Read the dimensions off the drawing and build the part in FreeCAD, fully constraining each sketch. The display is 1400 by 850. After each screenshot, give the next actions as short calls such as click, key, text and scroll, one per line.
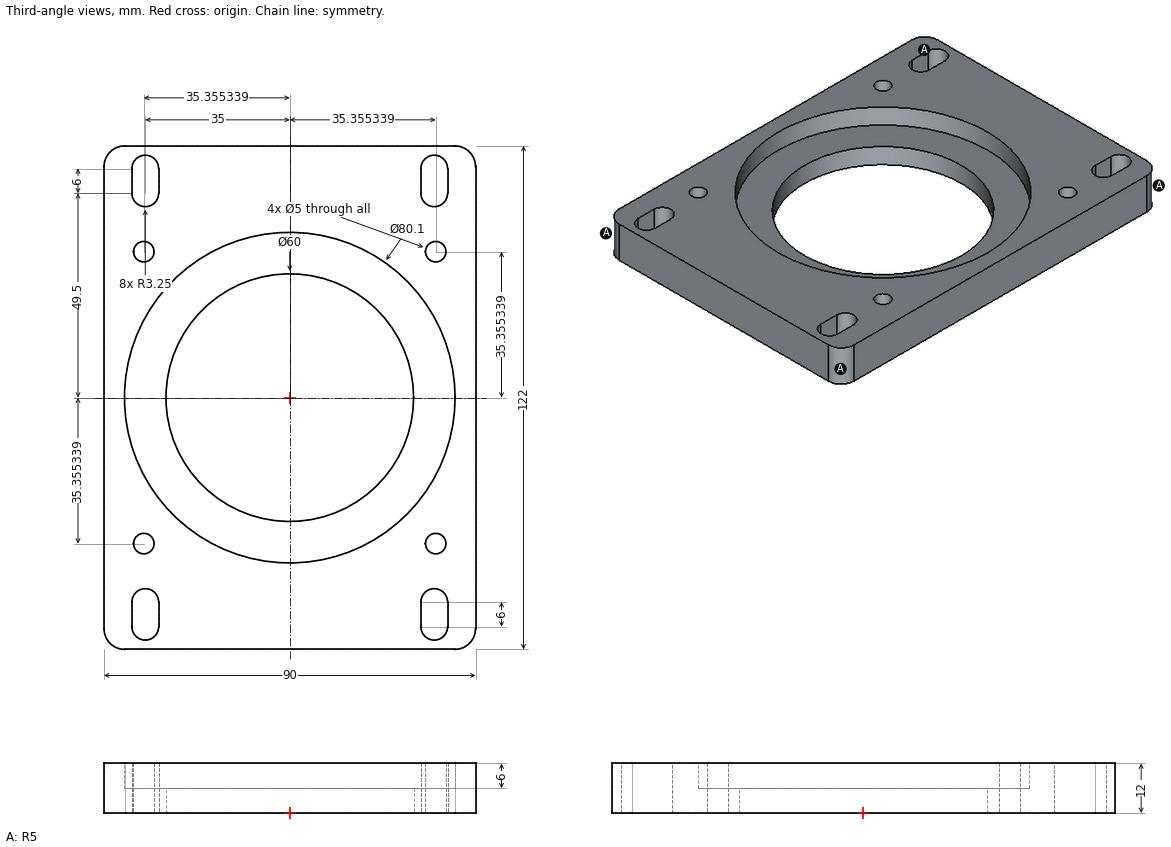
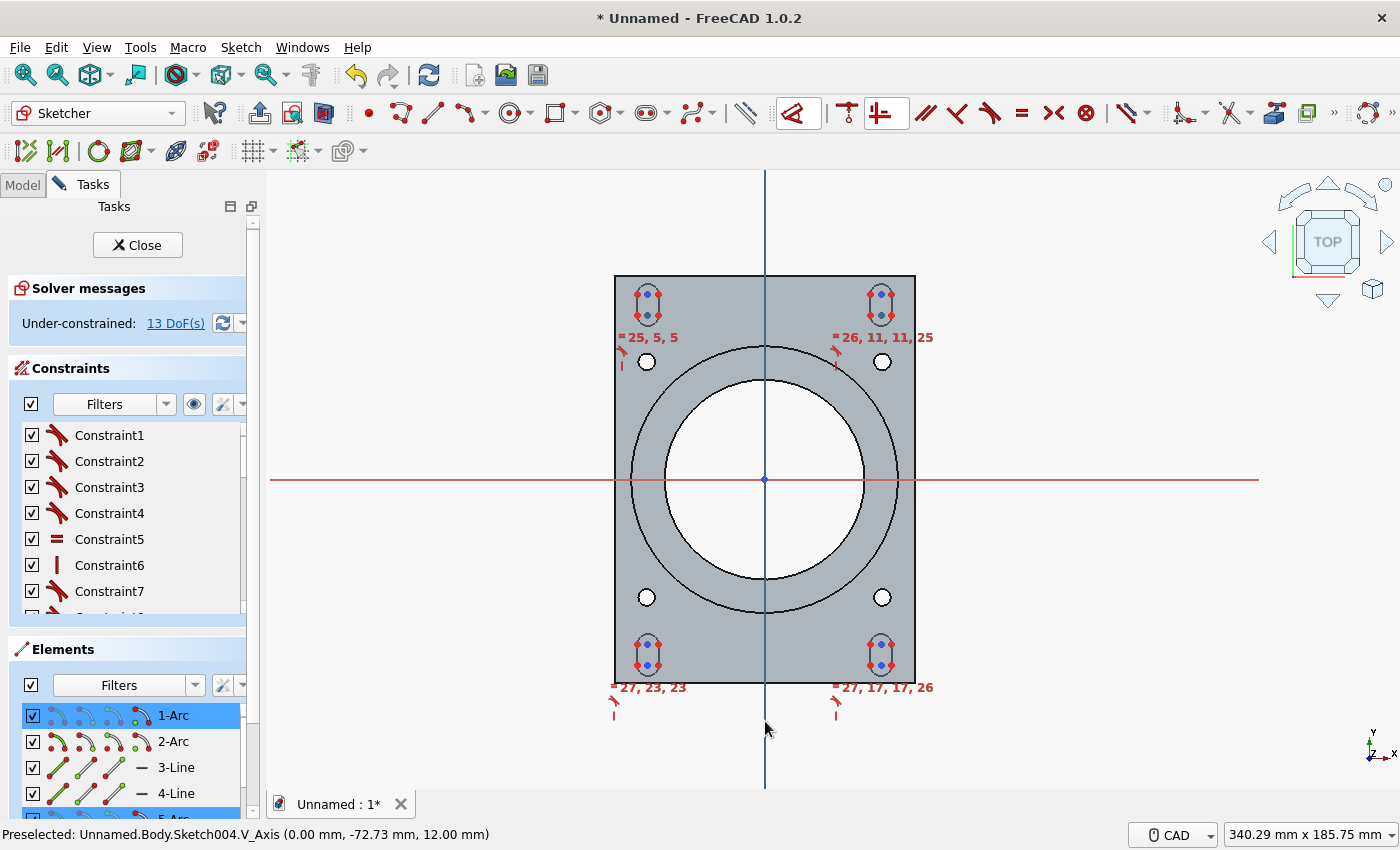
click(1054, 114)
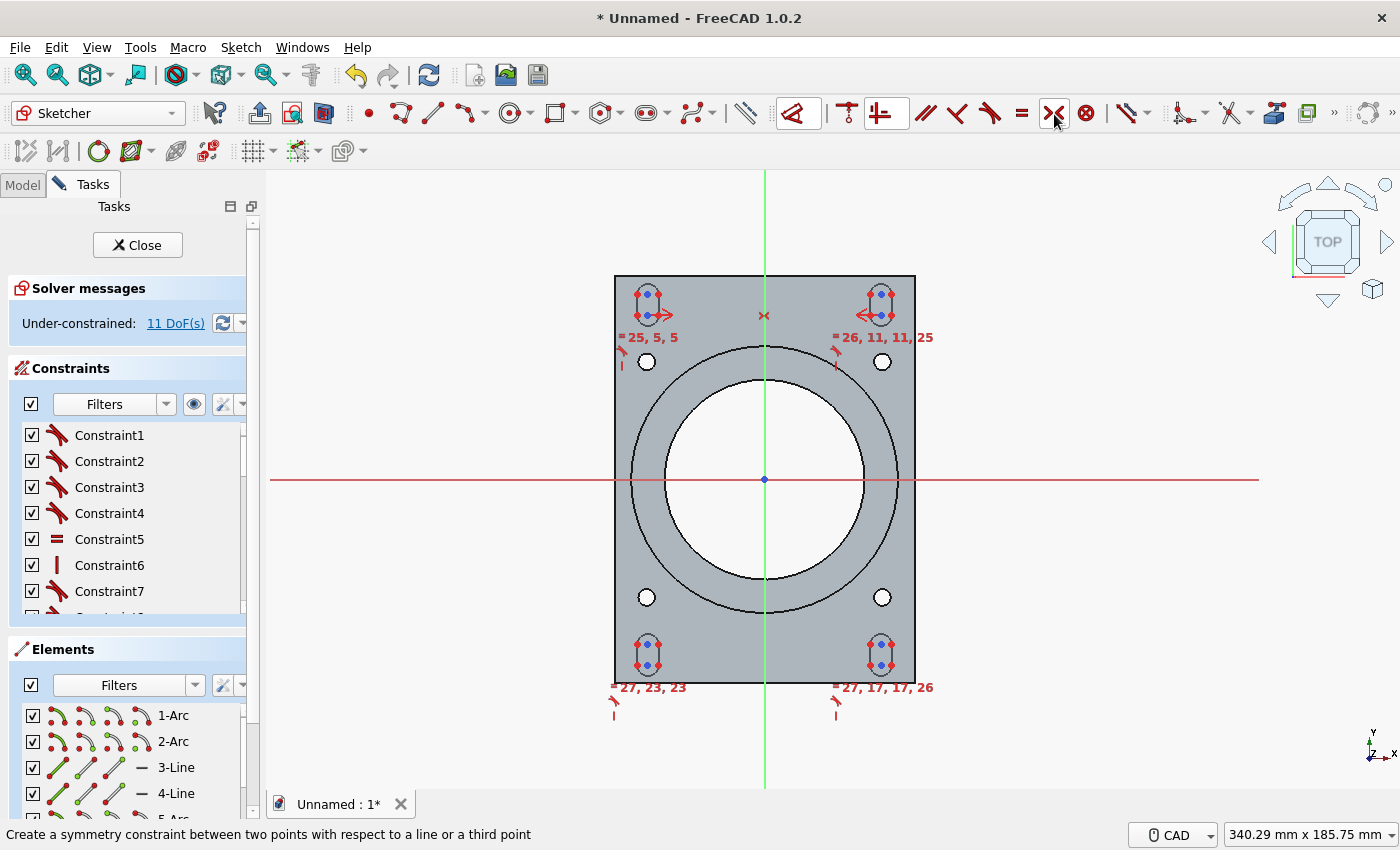
click(881, 295)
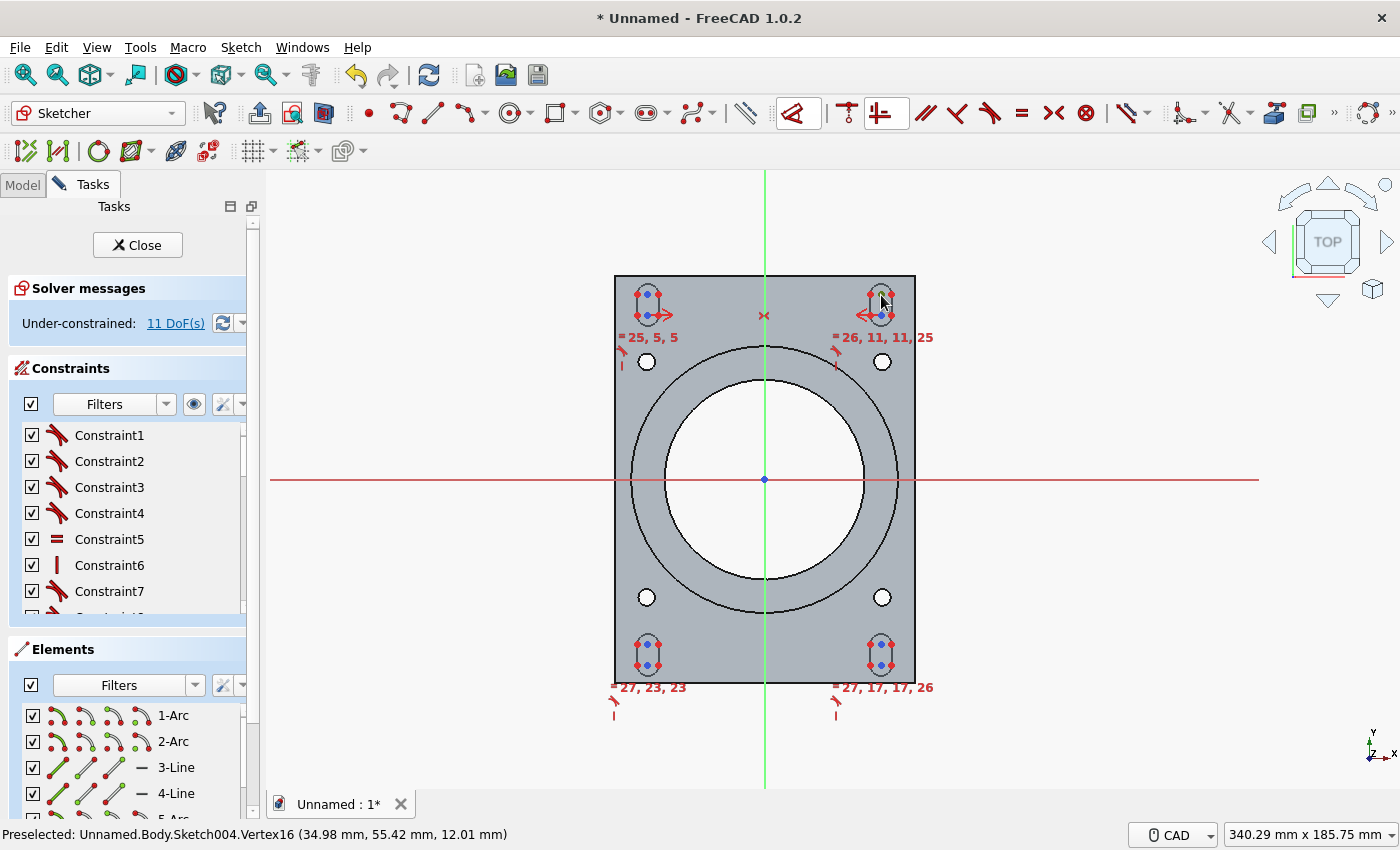
click(881, 665)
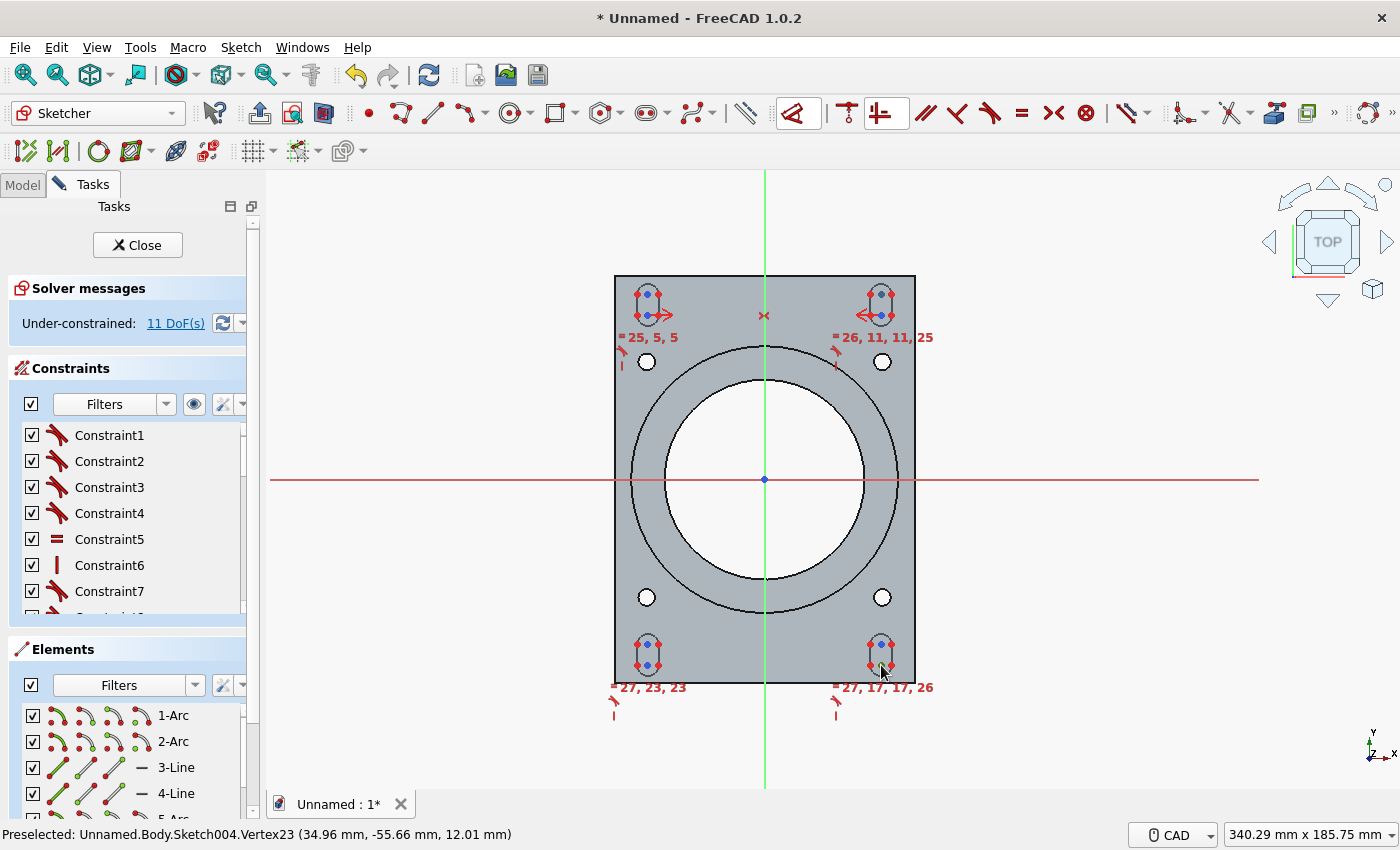
click(361, 480)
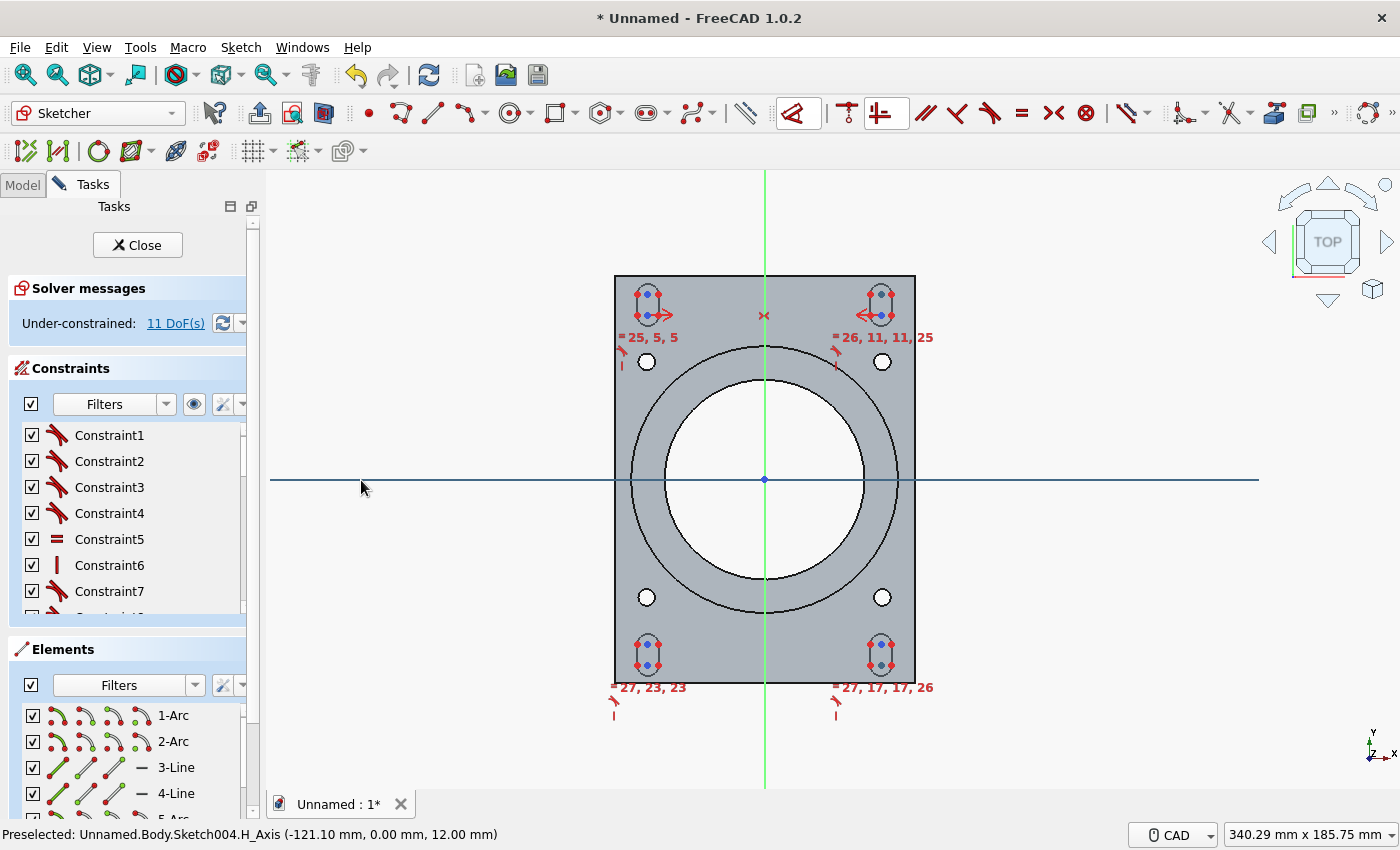
click(1054, 114)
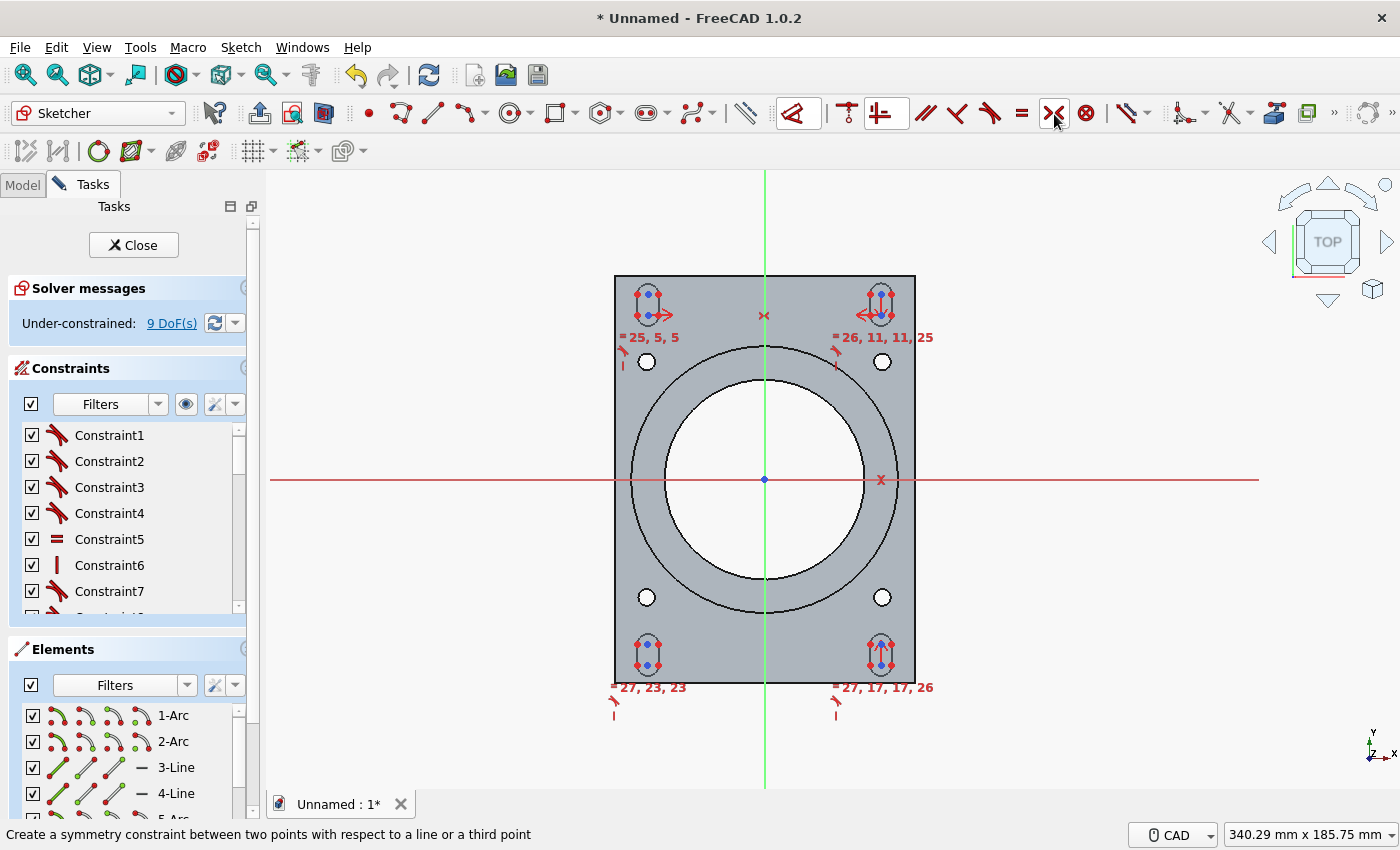
click(648, 295)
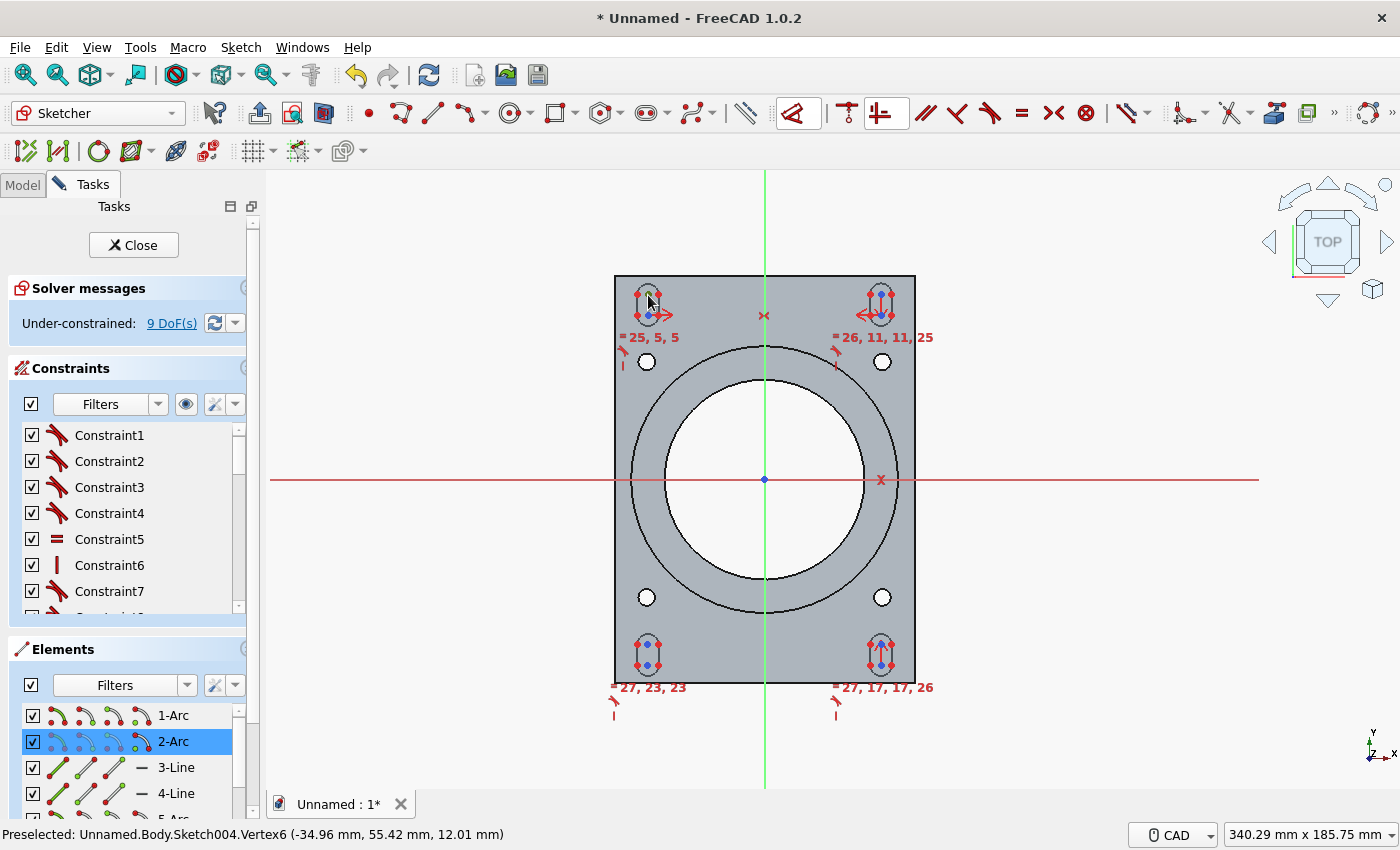
click(648, 665)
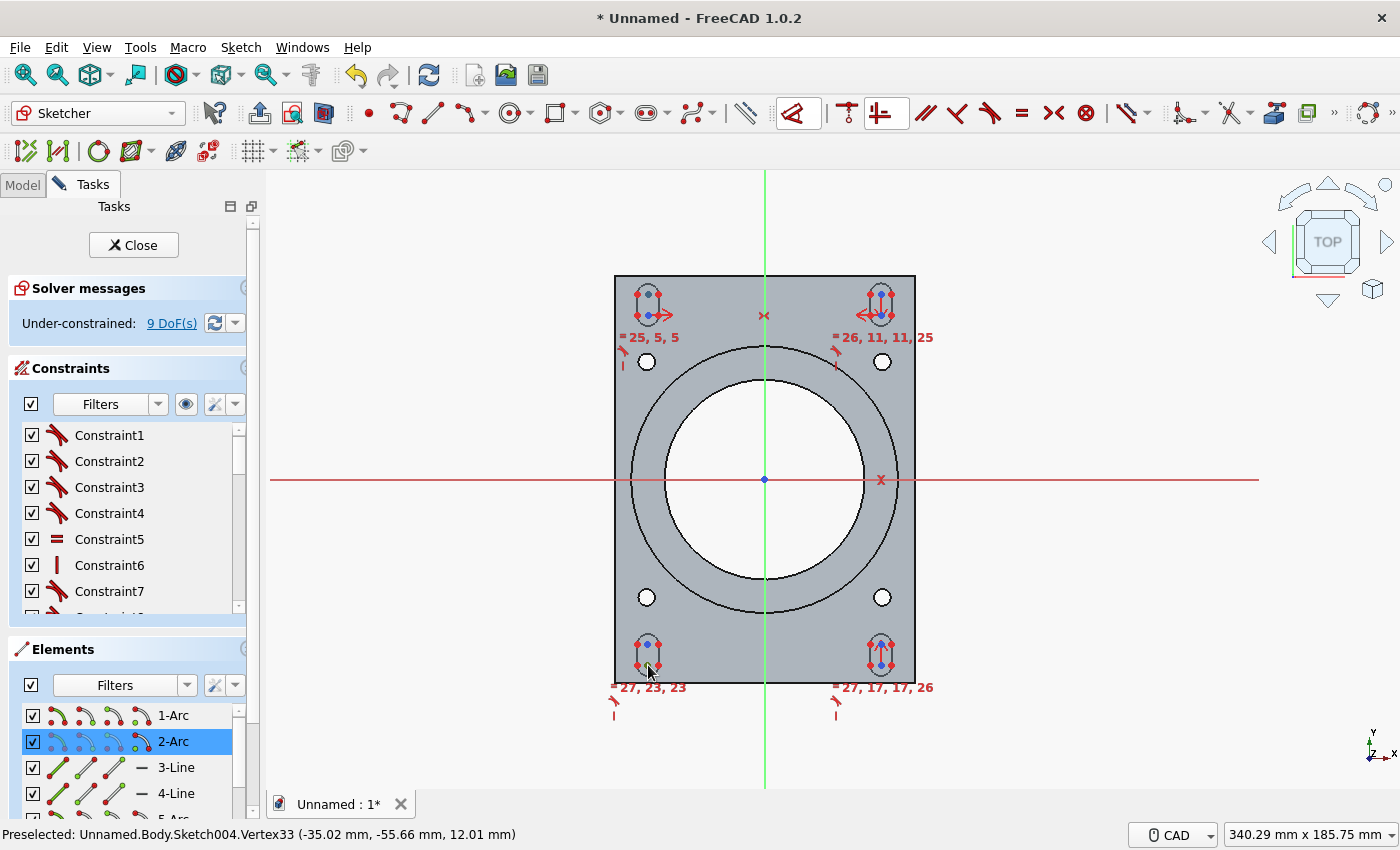
click(361, 480)